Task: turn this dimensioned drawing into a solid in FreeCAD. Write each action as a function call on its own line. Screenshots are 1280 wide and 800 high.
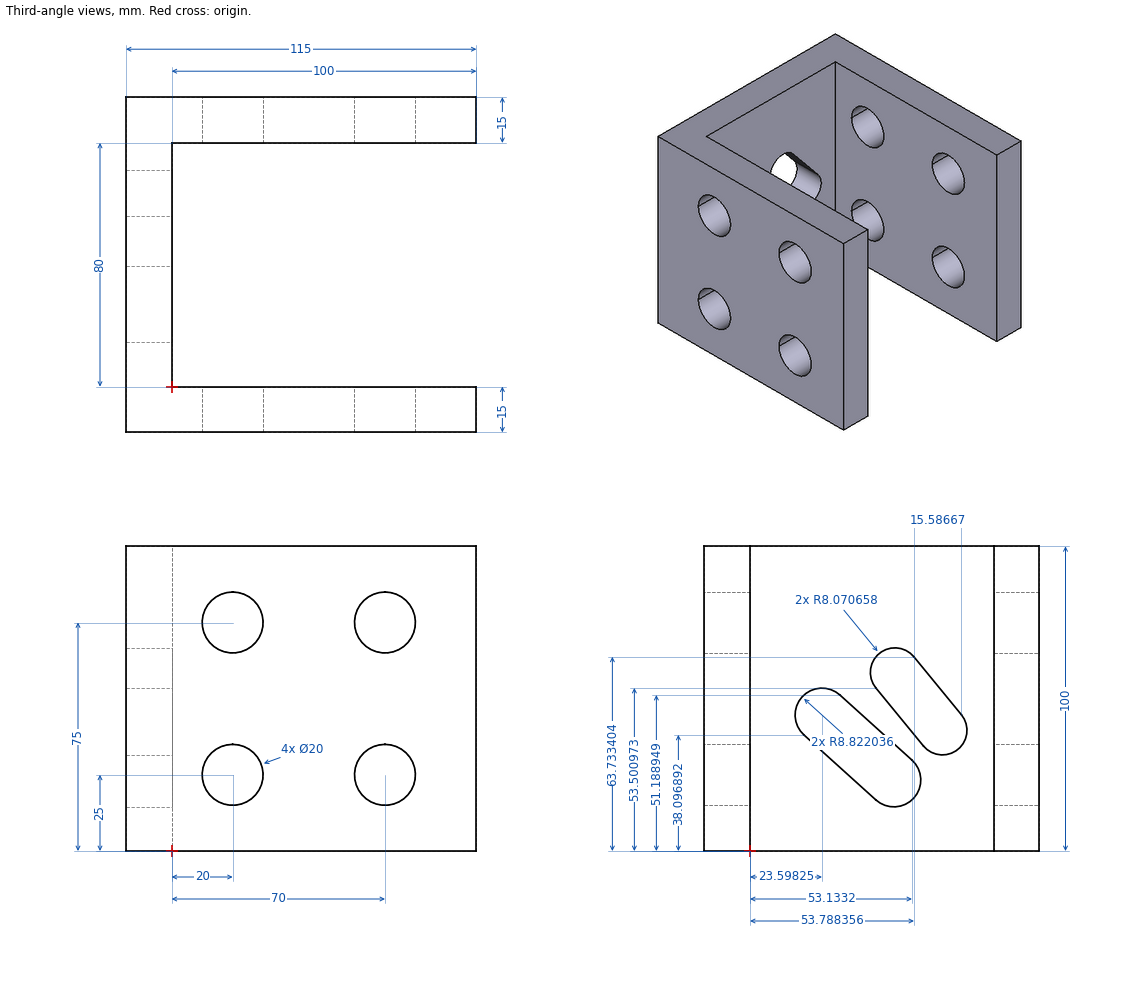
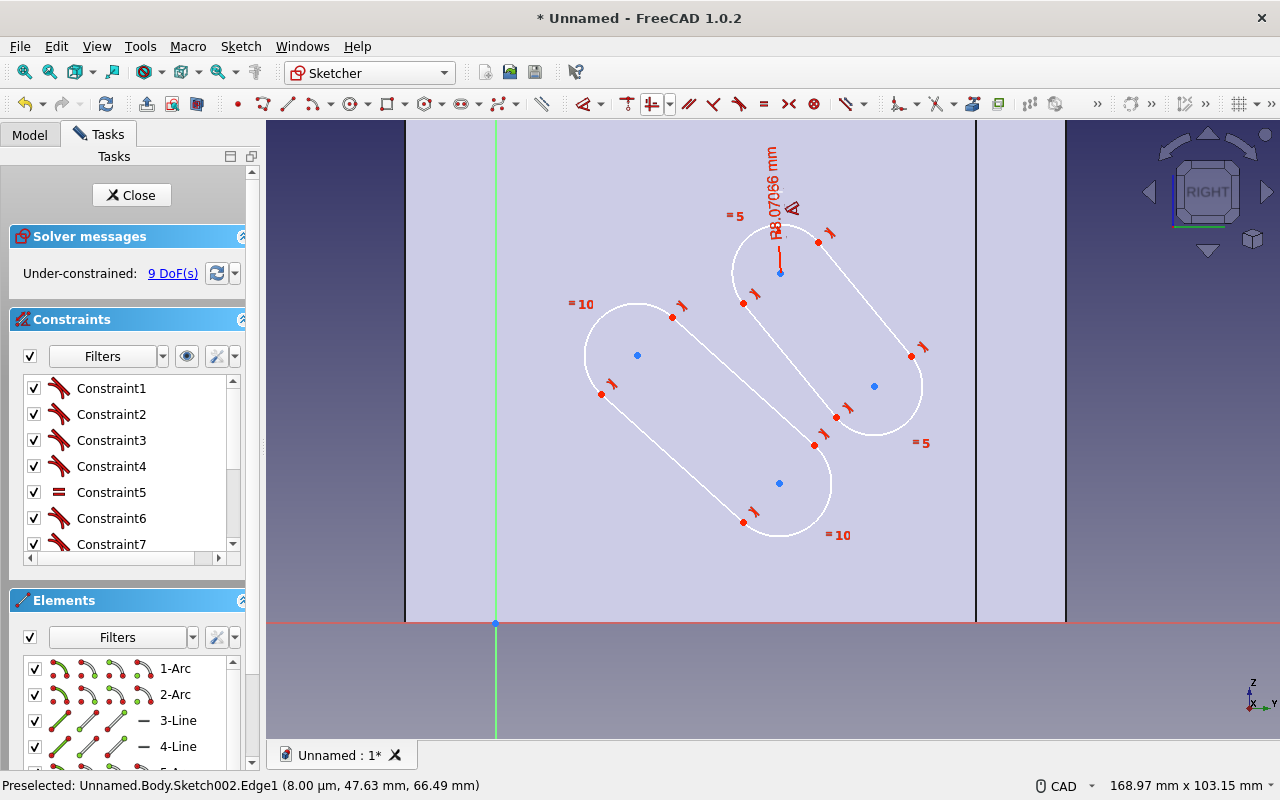
click(626, 305)
click(619, 274)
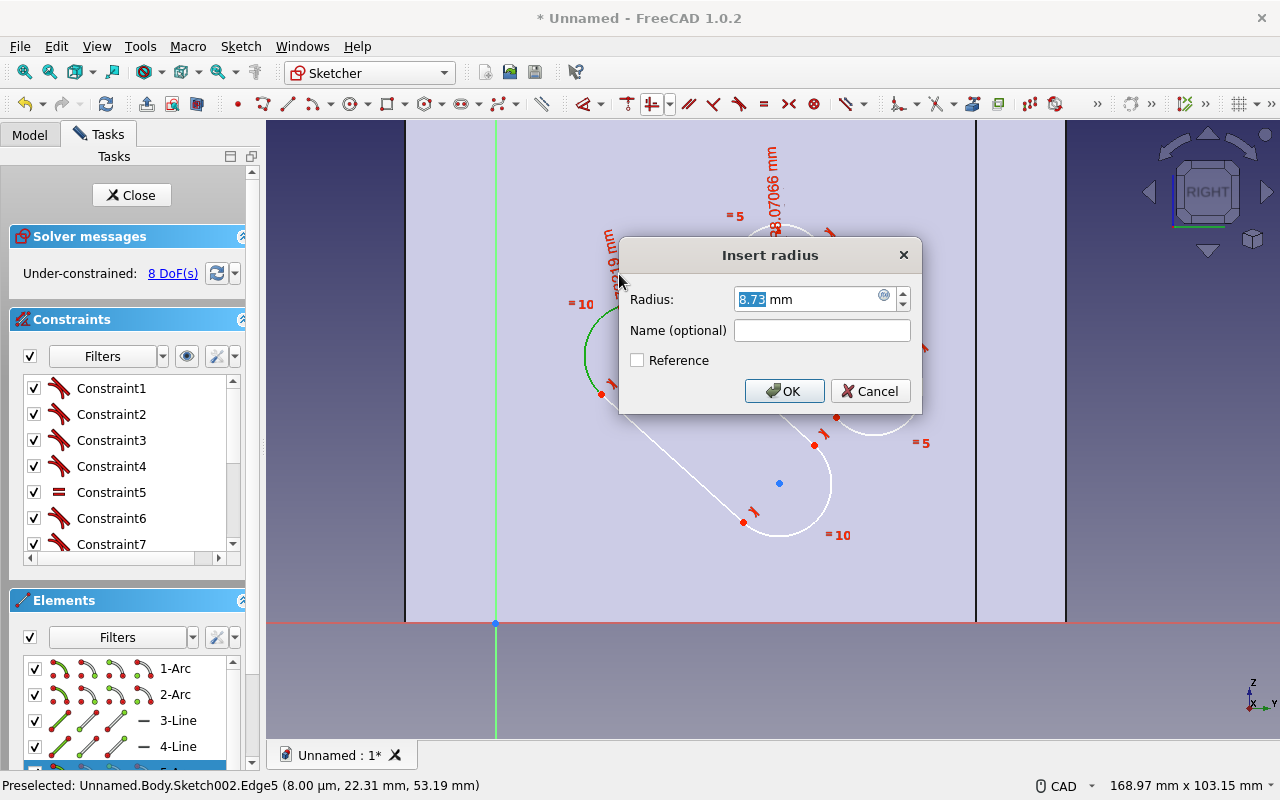
text(8.822036)
key(Return)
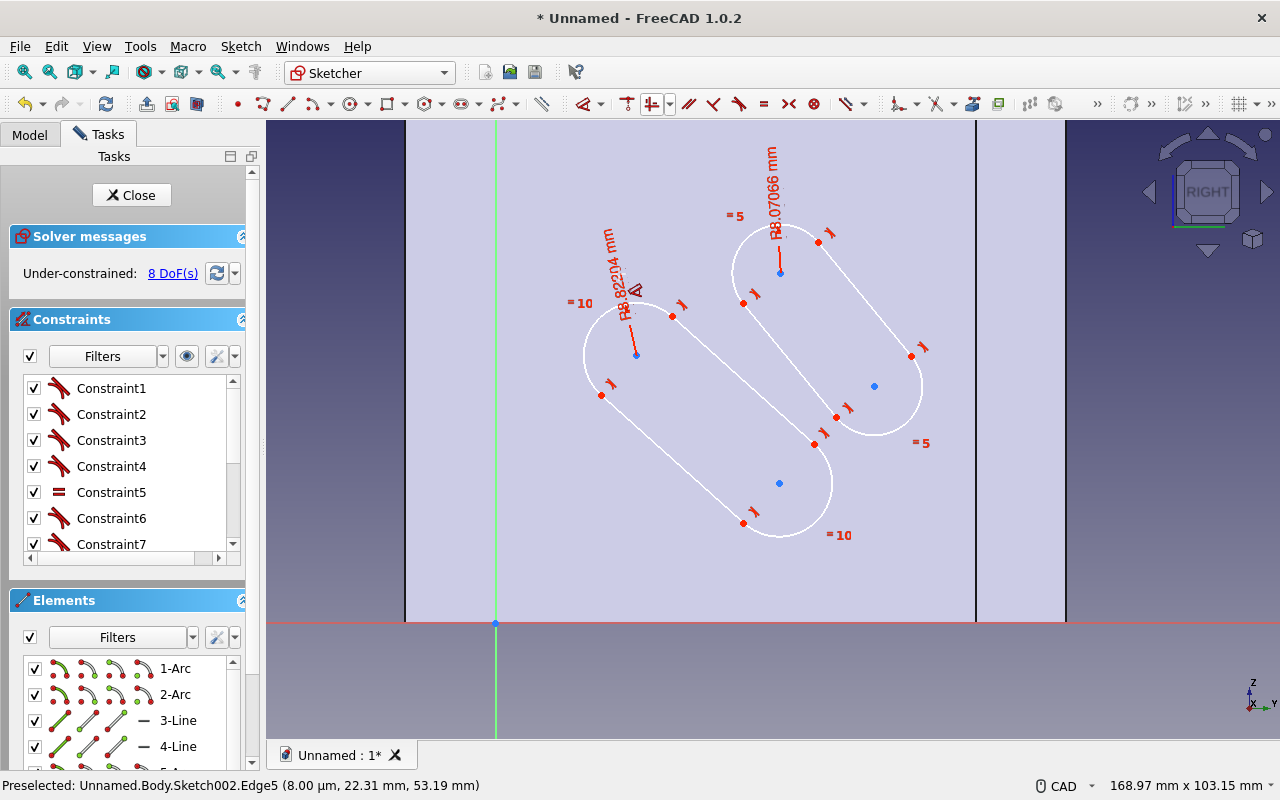
click(815, 444)
click(655, 657)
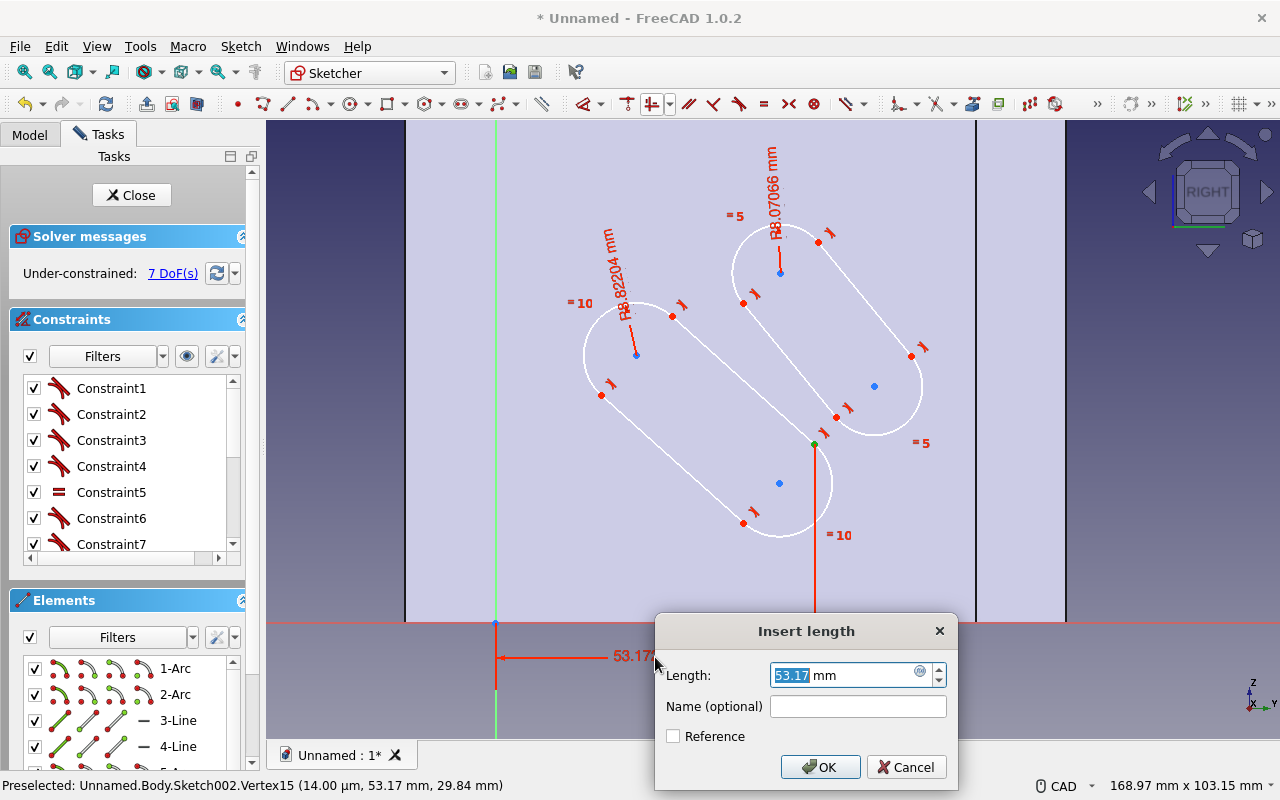
text(53.1332)
key(Return)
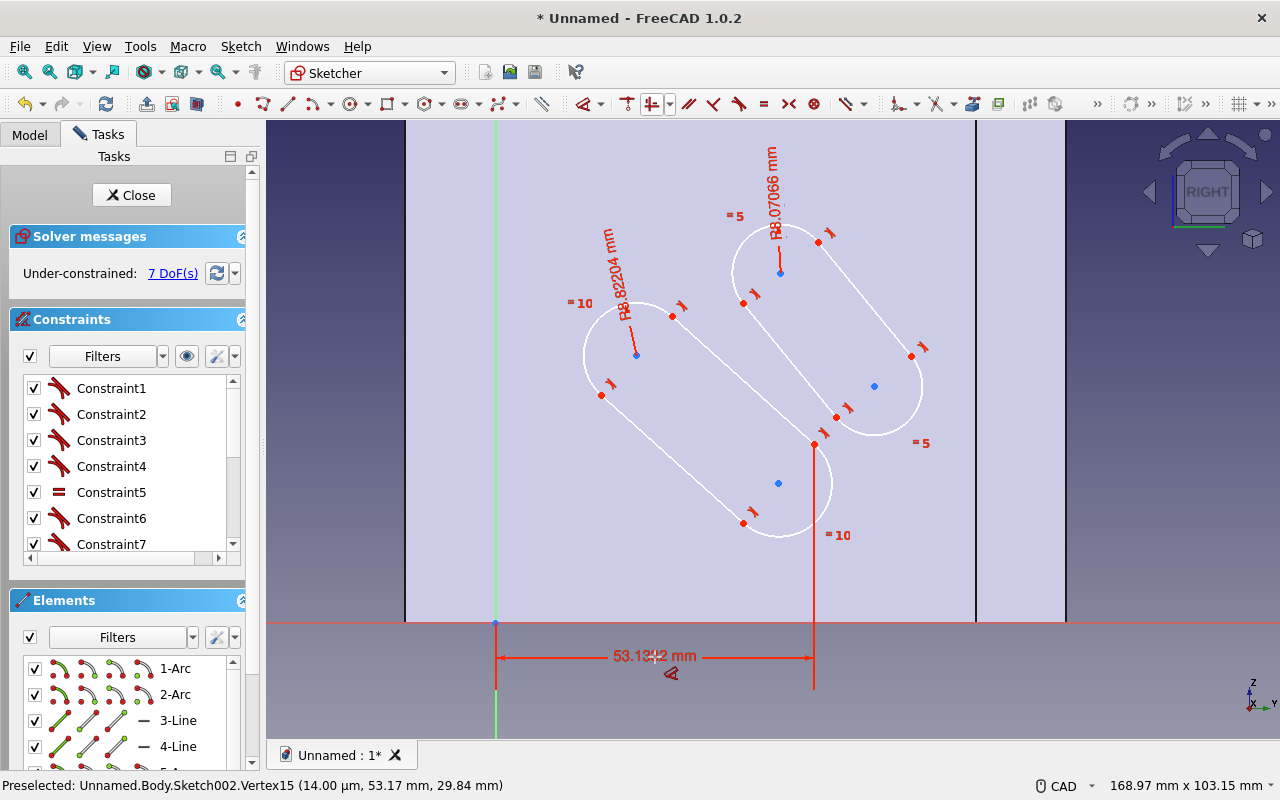
click(846, 277)
click(865, 208)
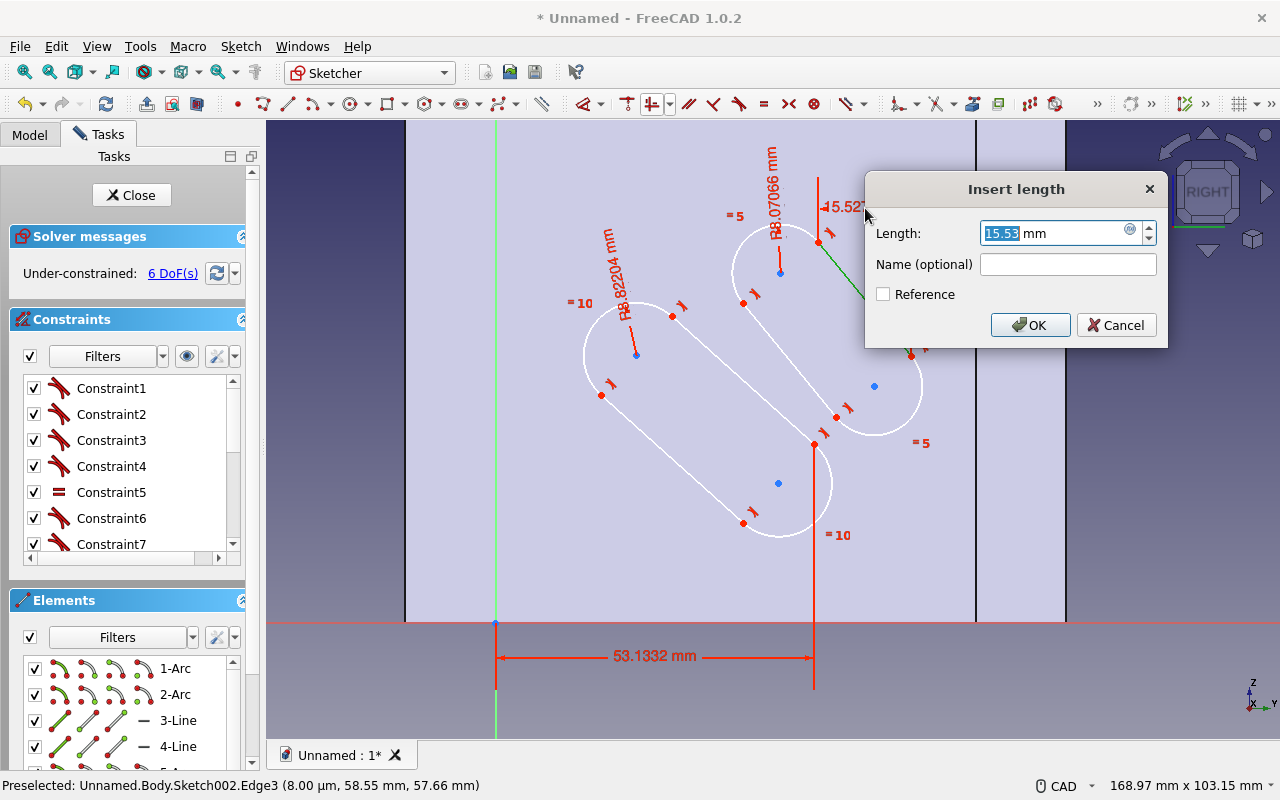
text(15.58667)
key(Return)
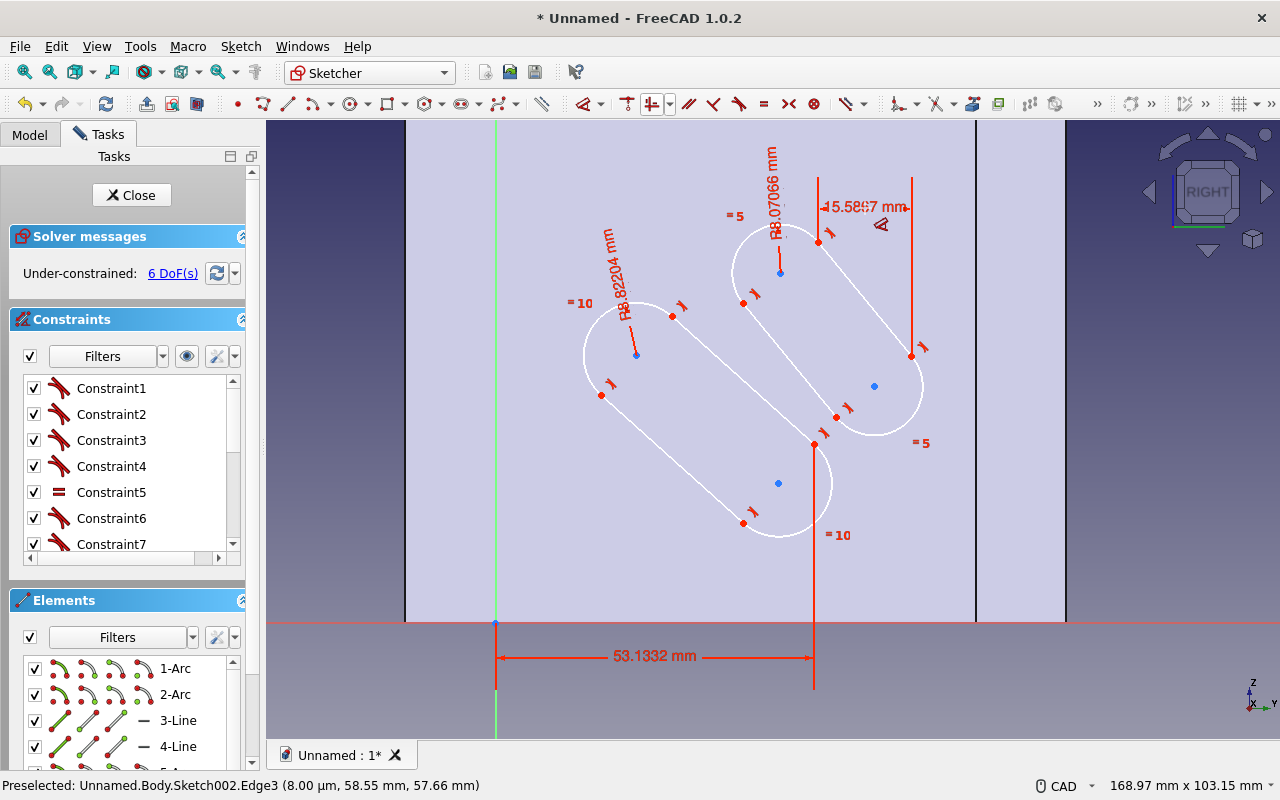
click(637, 356)
click(566, 657)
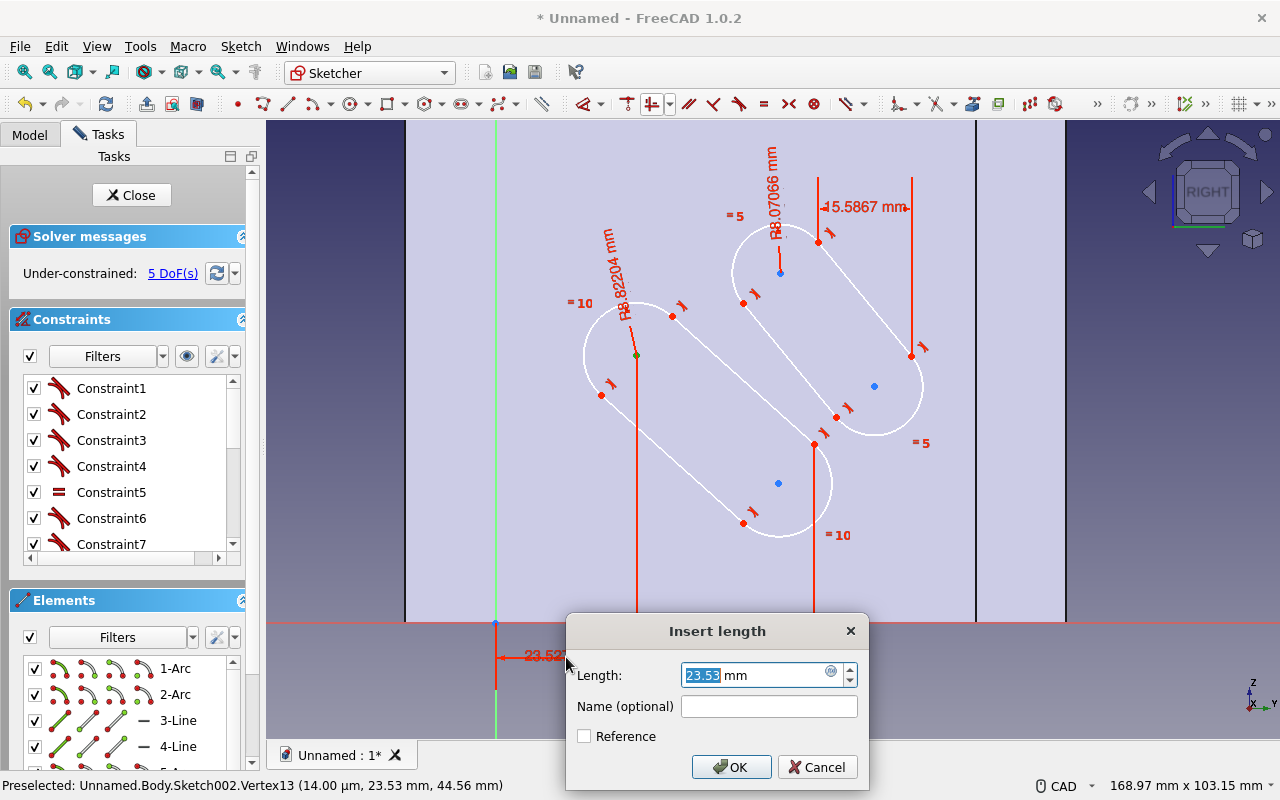
text(23.59825)
key(Return)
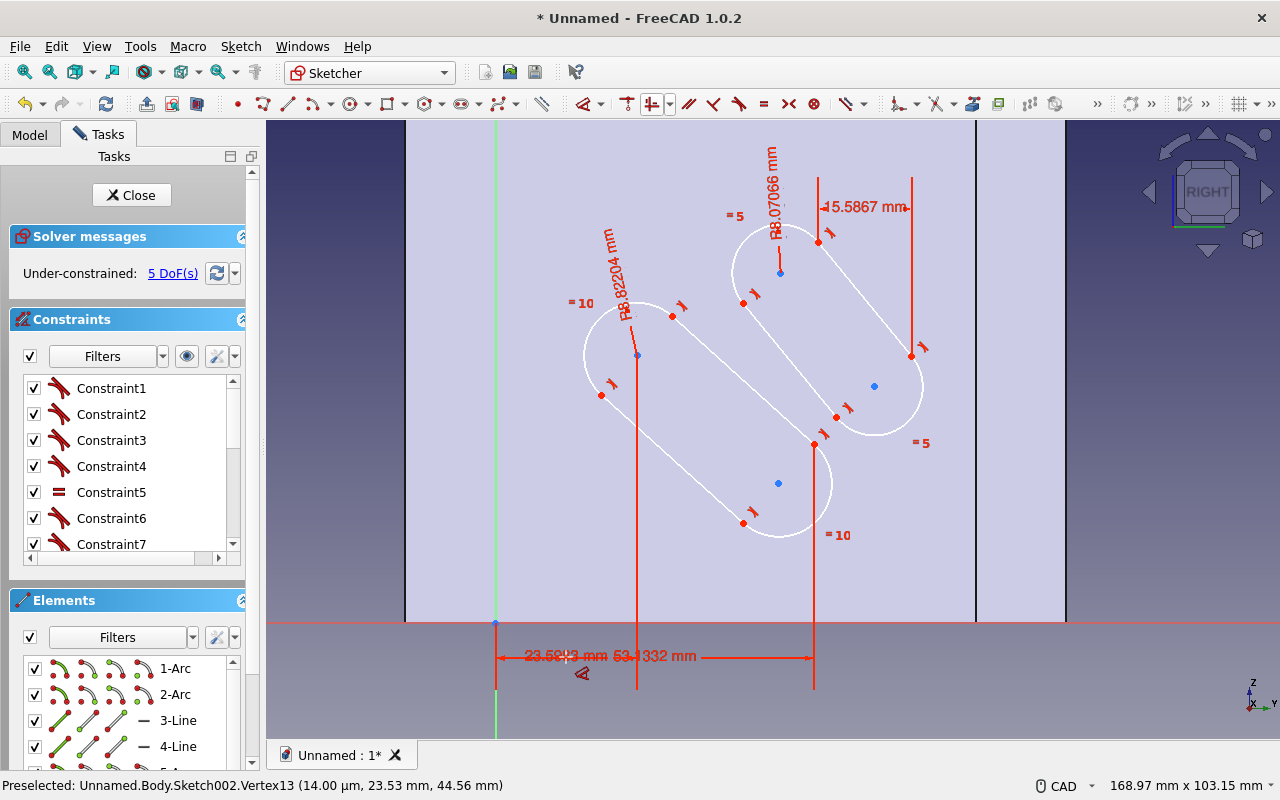
click(818, 242)
click(731, 657)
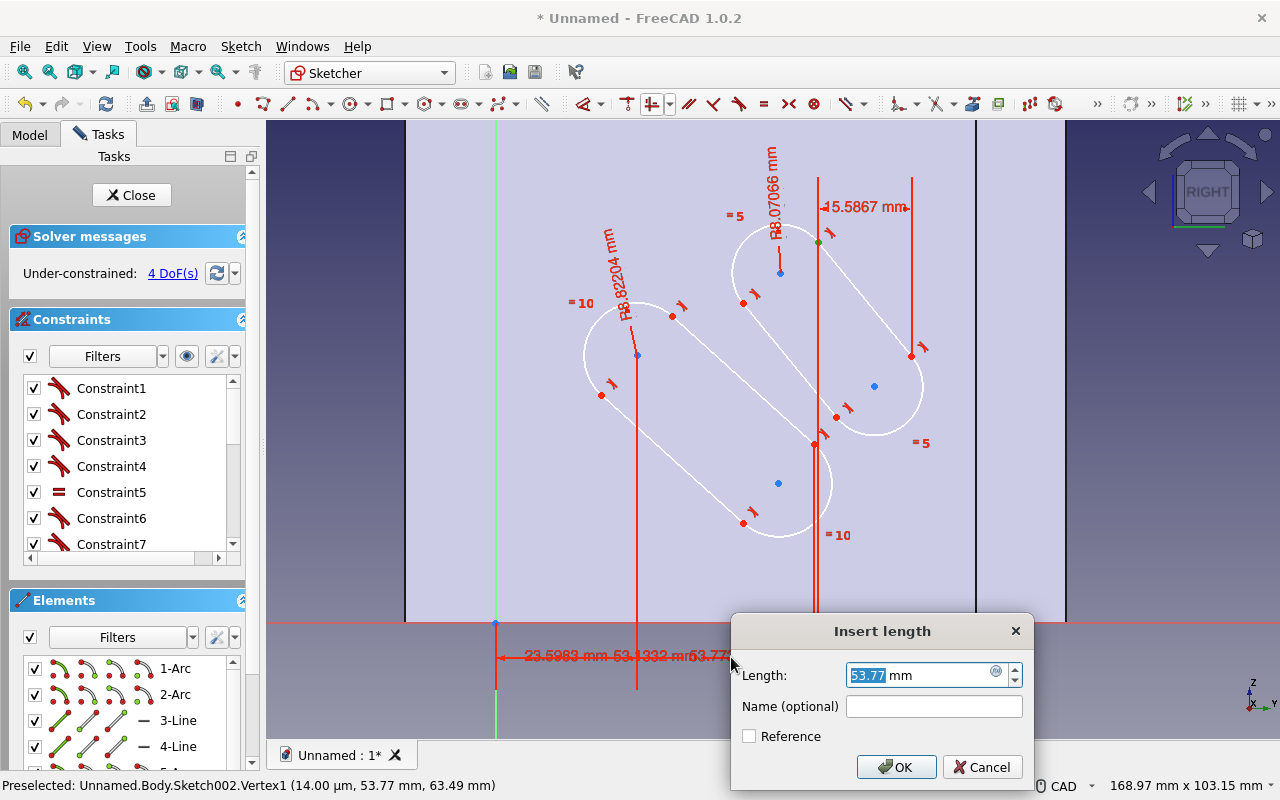
text(53.788356)
key(Return)